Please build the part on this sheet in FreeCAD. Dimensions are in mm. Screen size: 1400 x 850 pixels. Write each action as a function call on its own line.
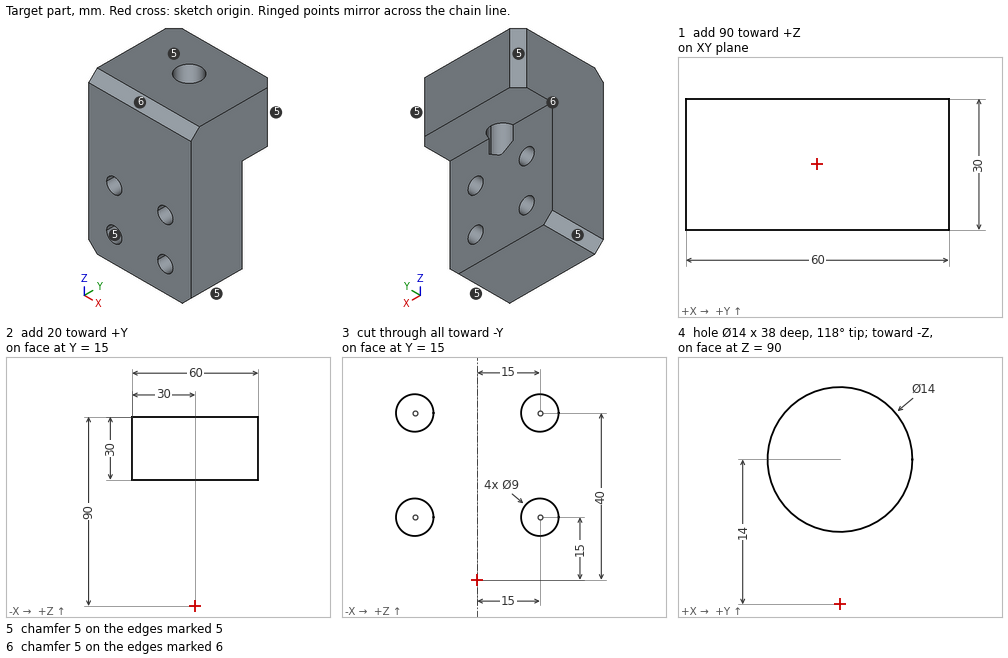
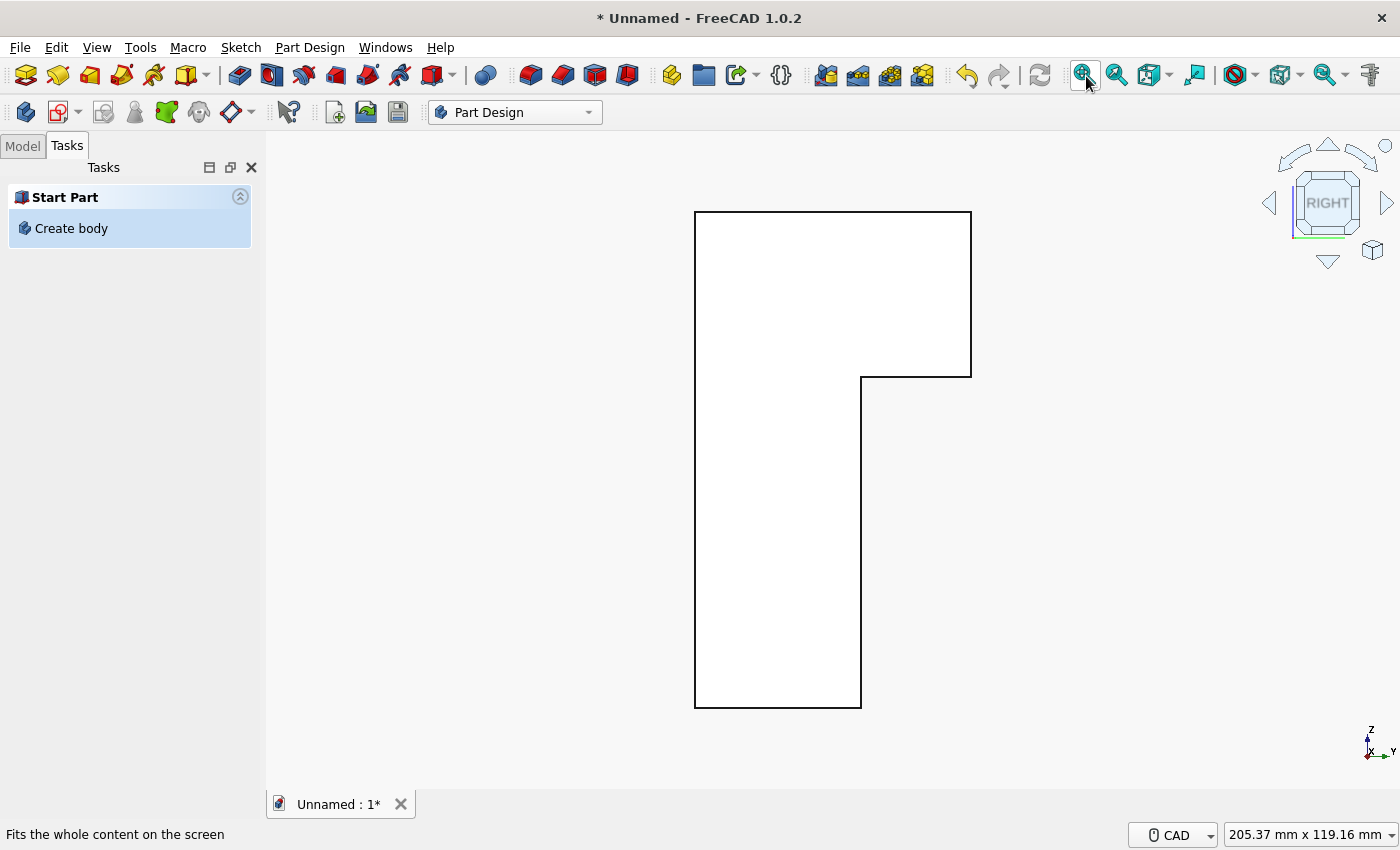
click(971, 293)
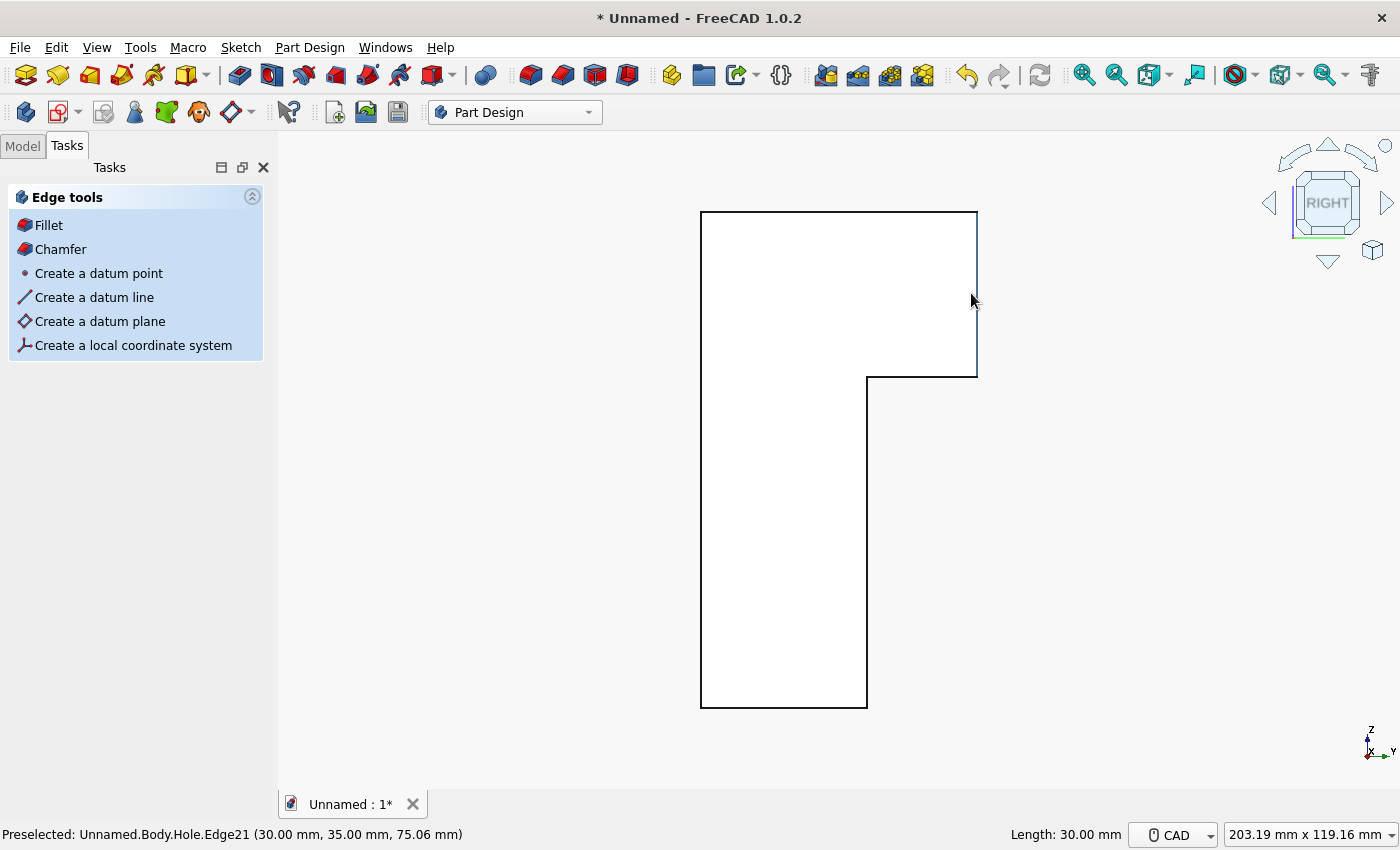
click(784, 707, ctrl)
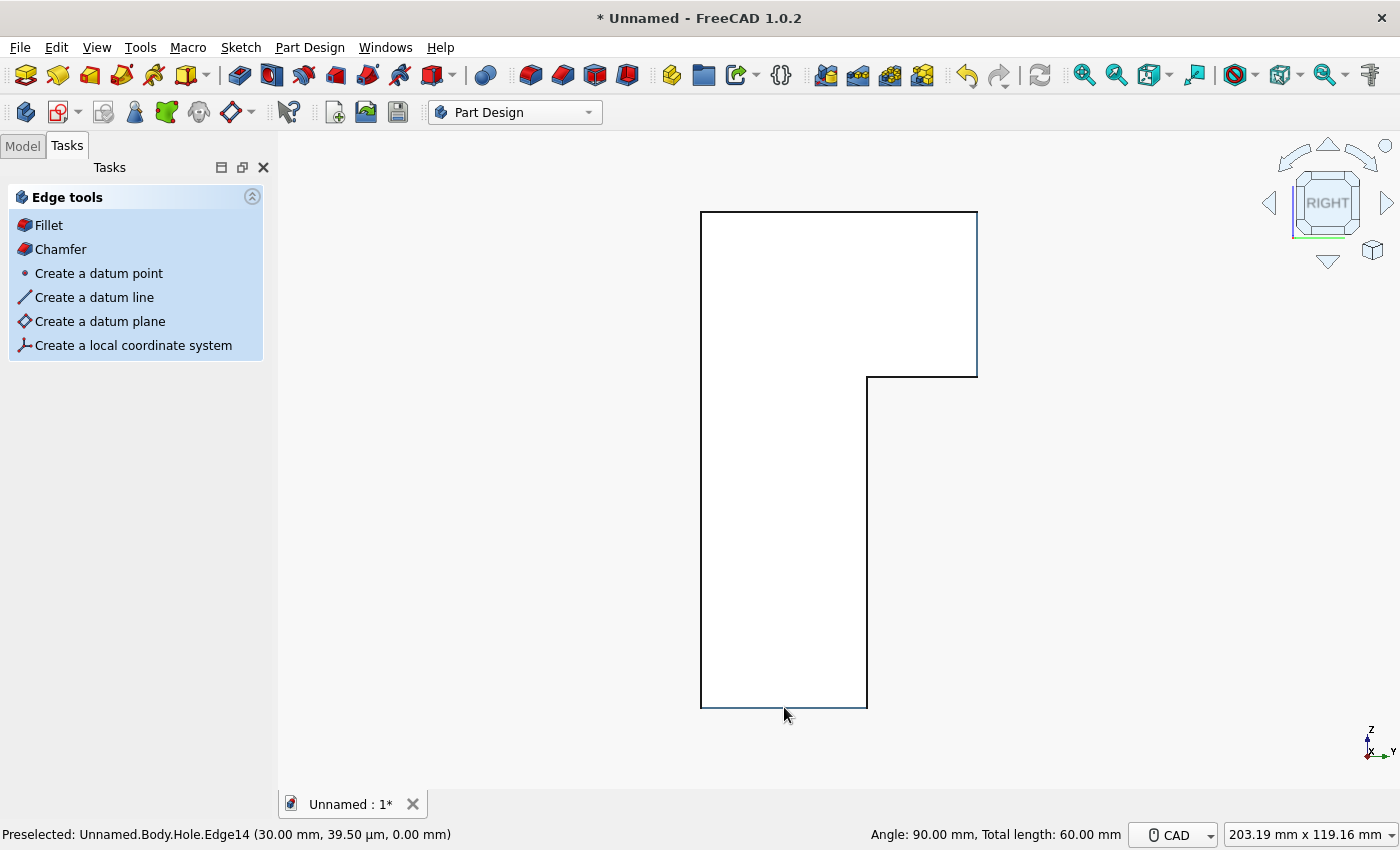
key(5)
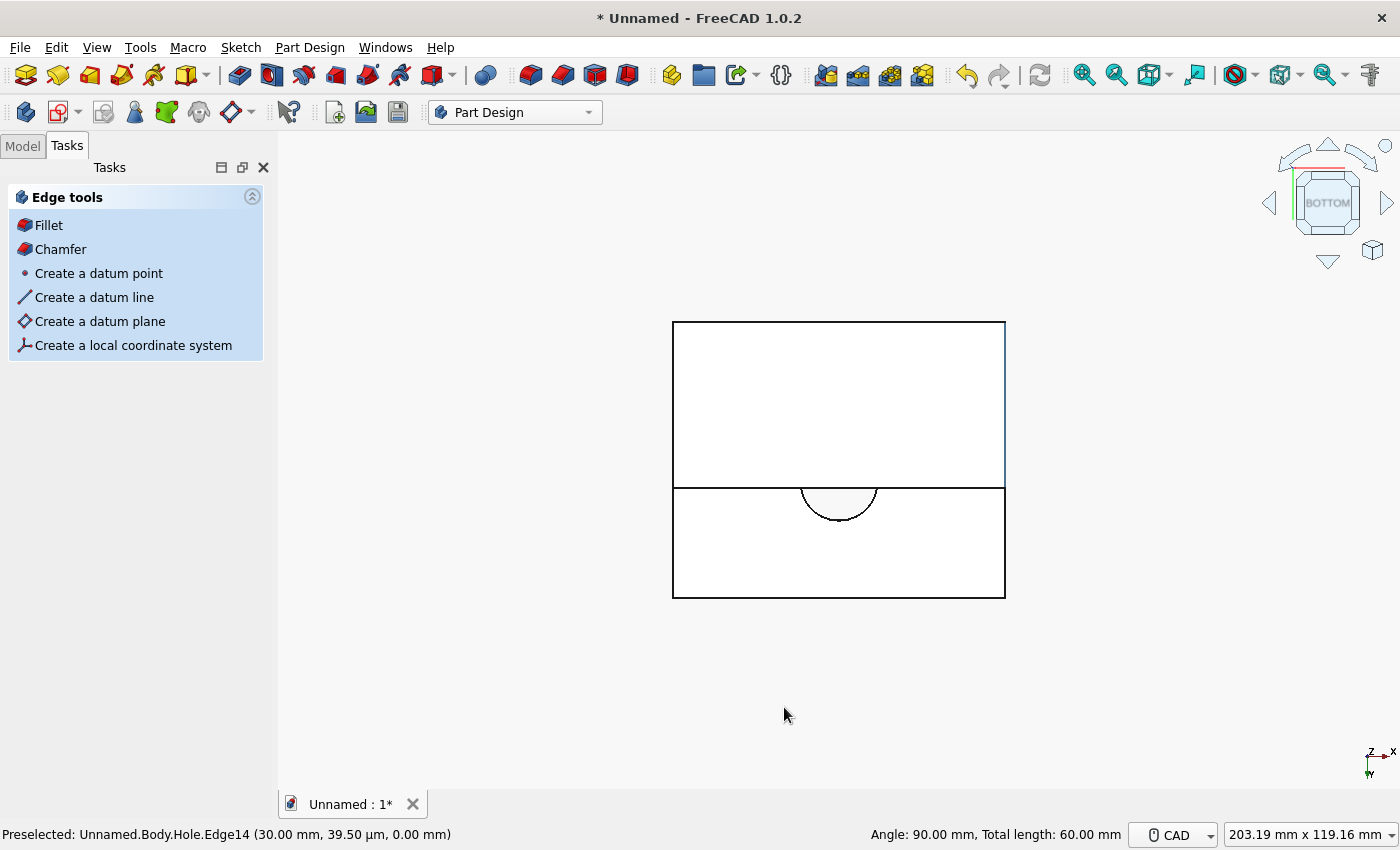
click(1086, 76)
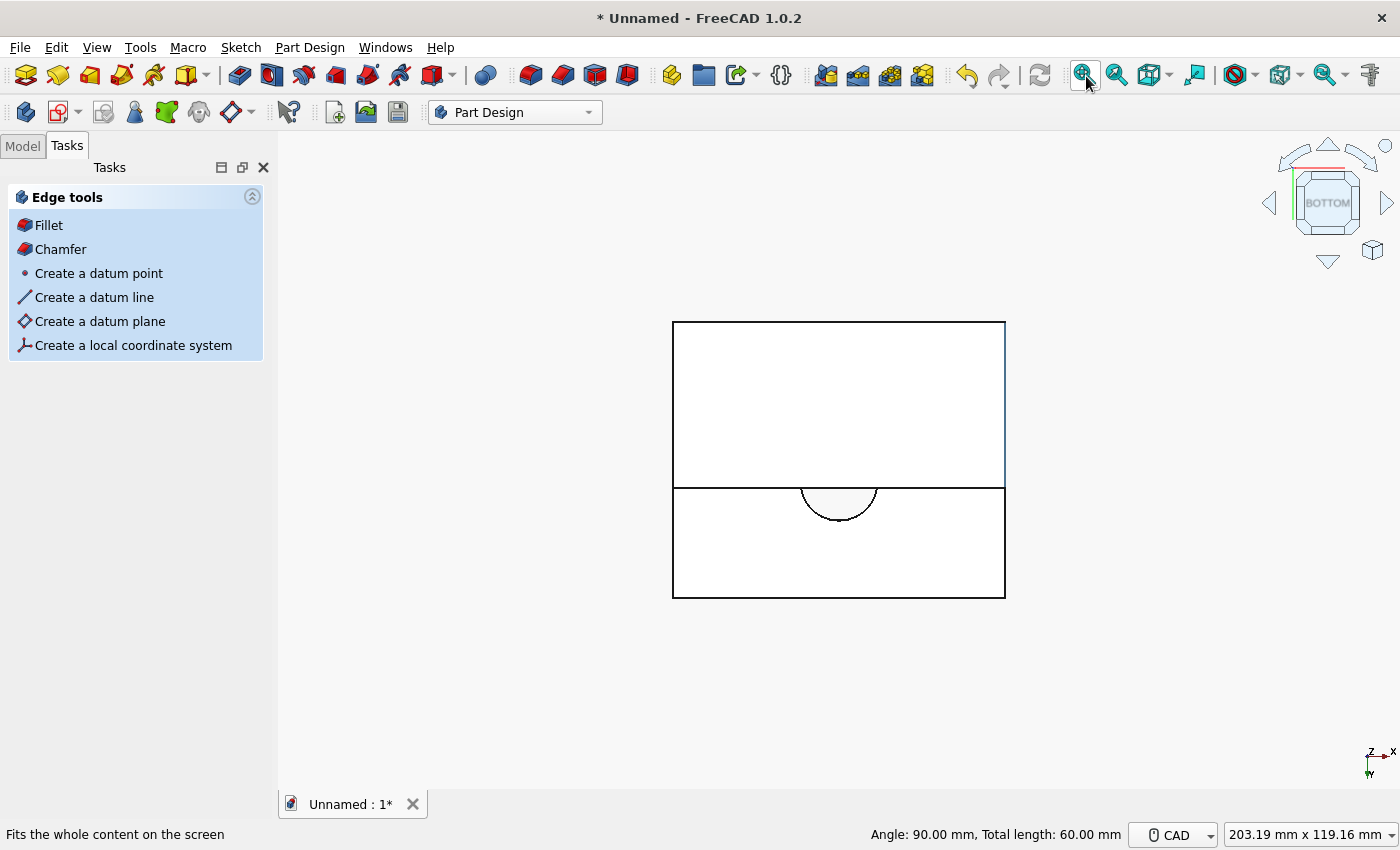
click(673, 404, ctrl)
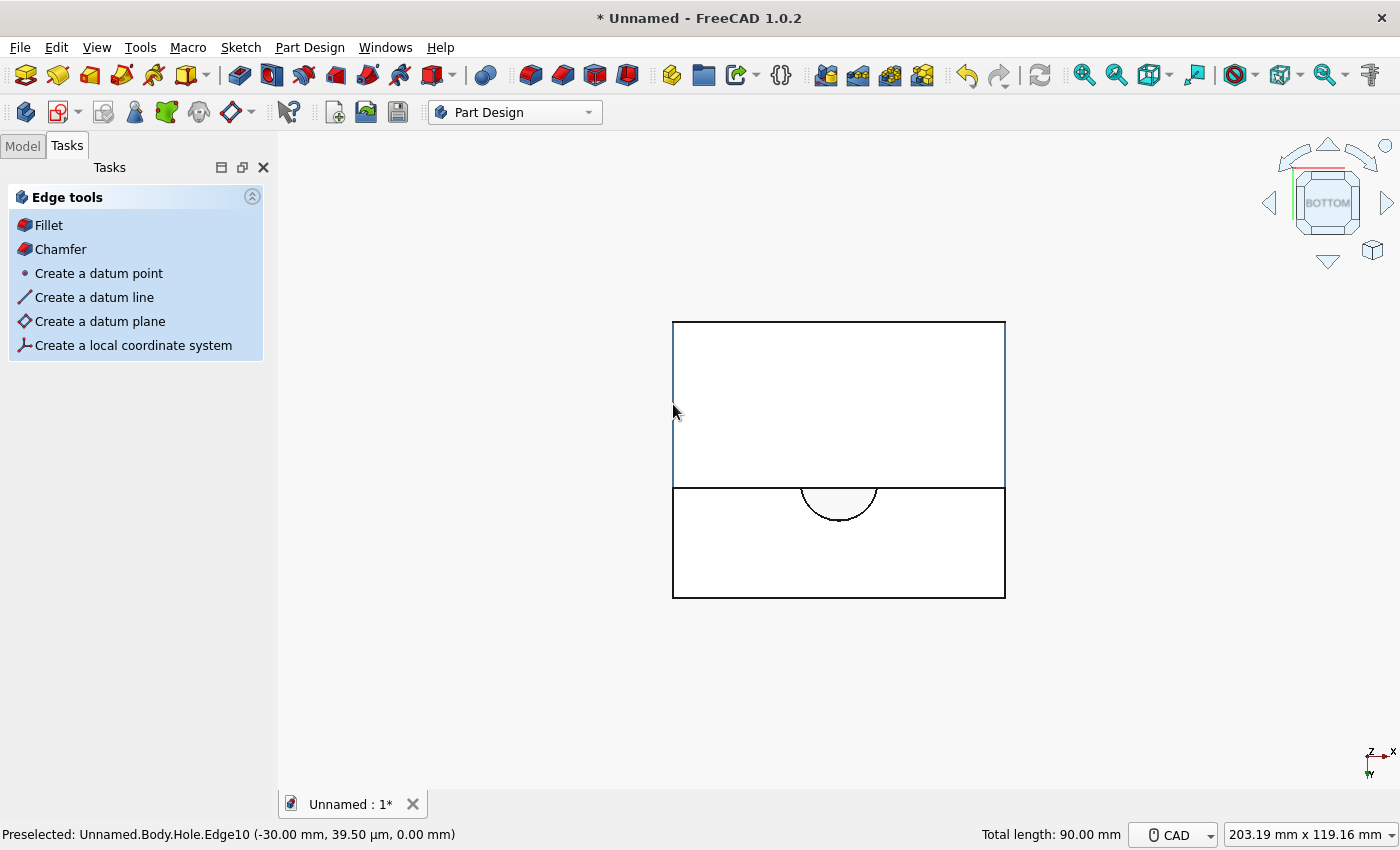
key(4)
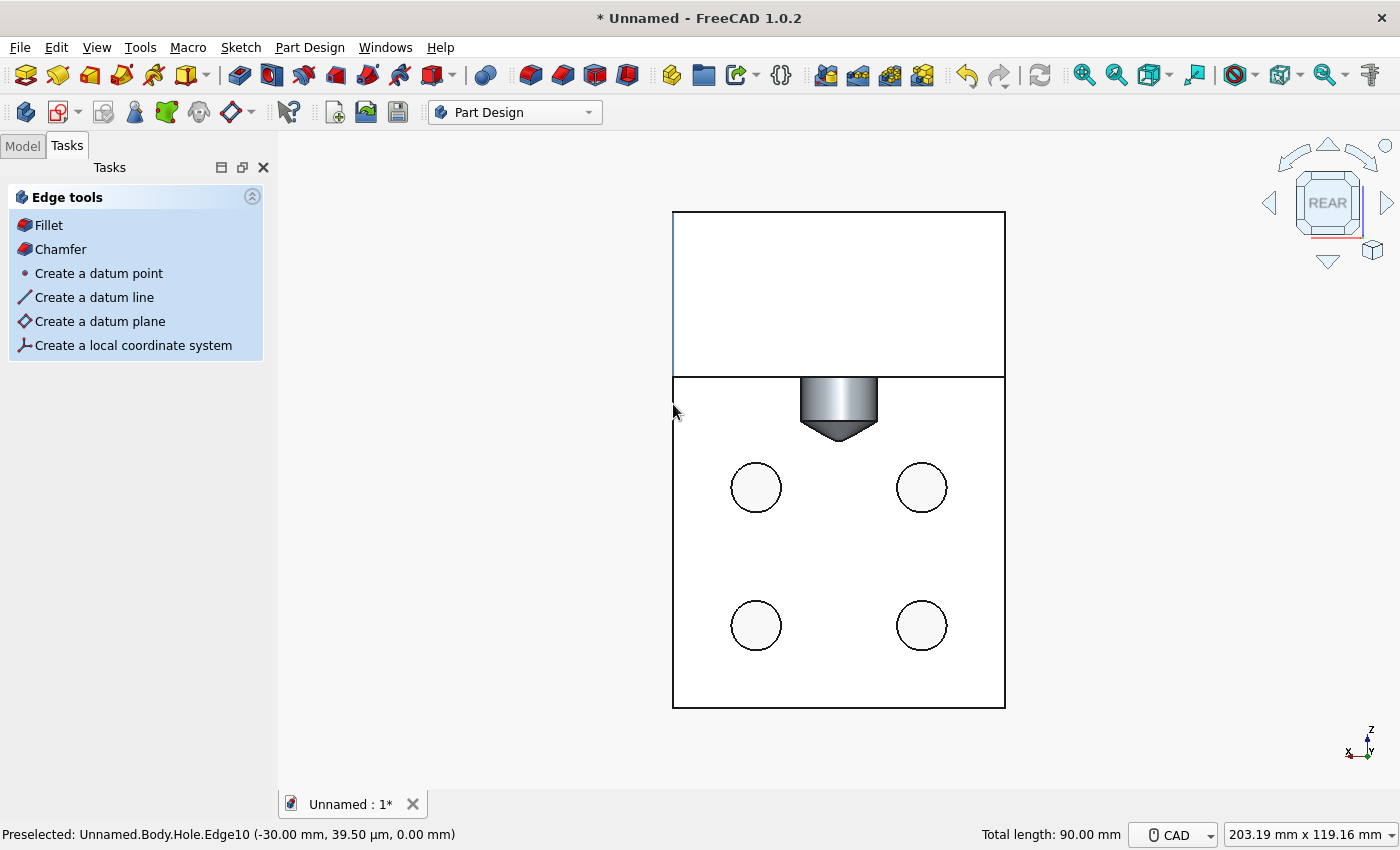
click(1005, 293, ctrl)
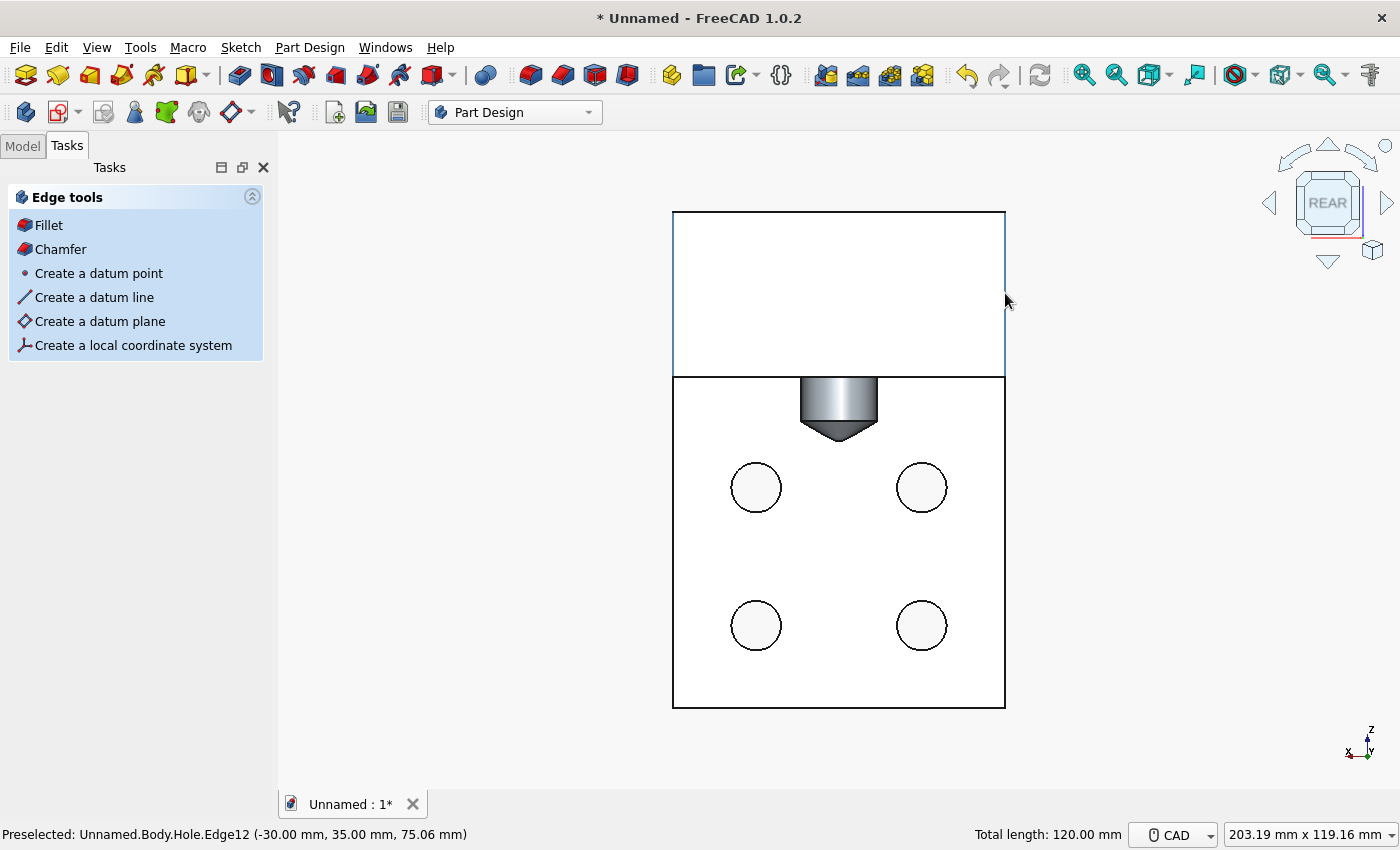
click(564, 76)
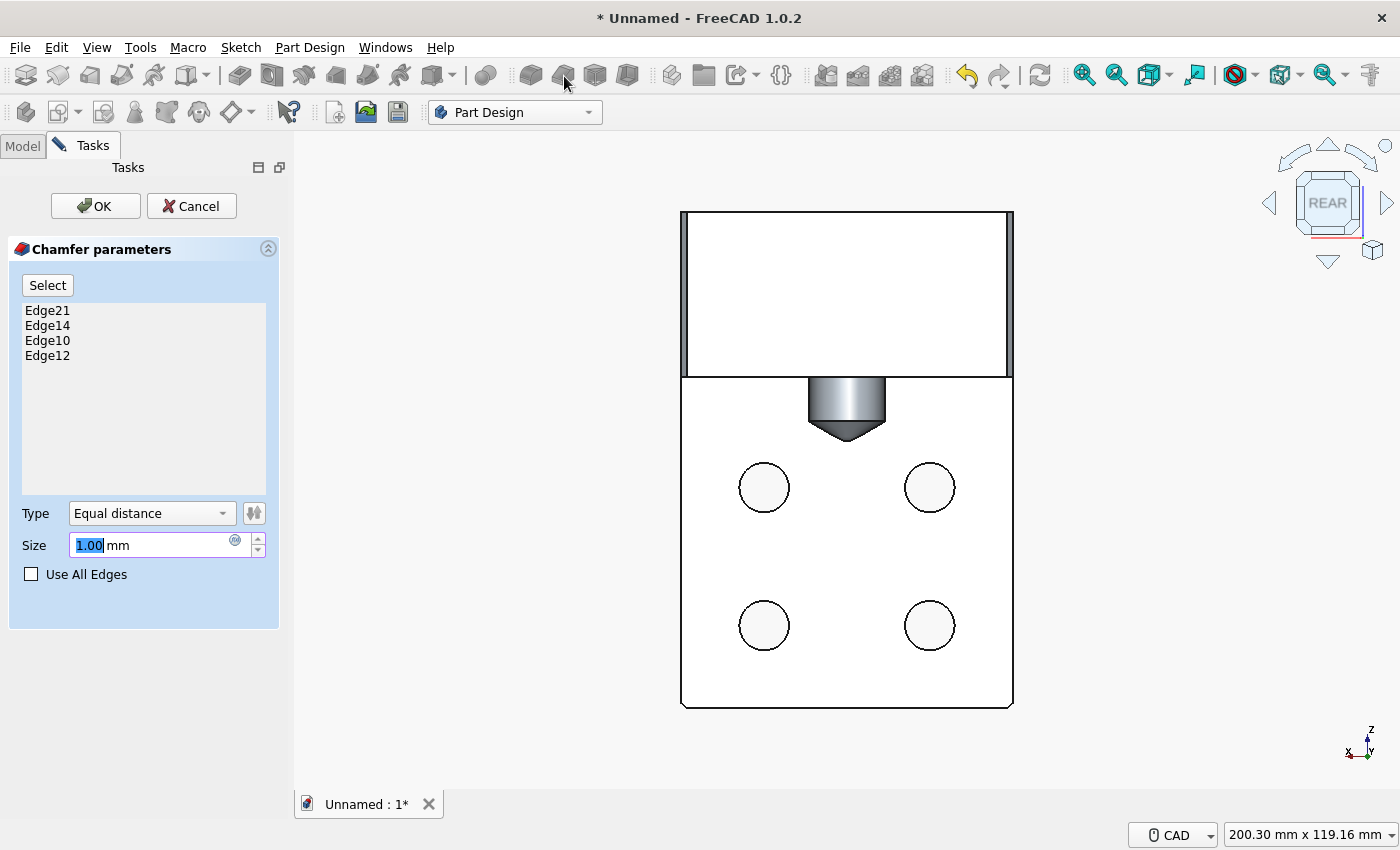
text(5)
key(Tab)